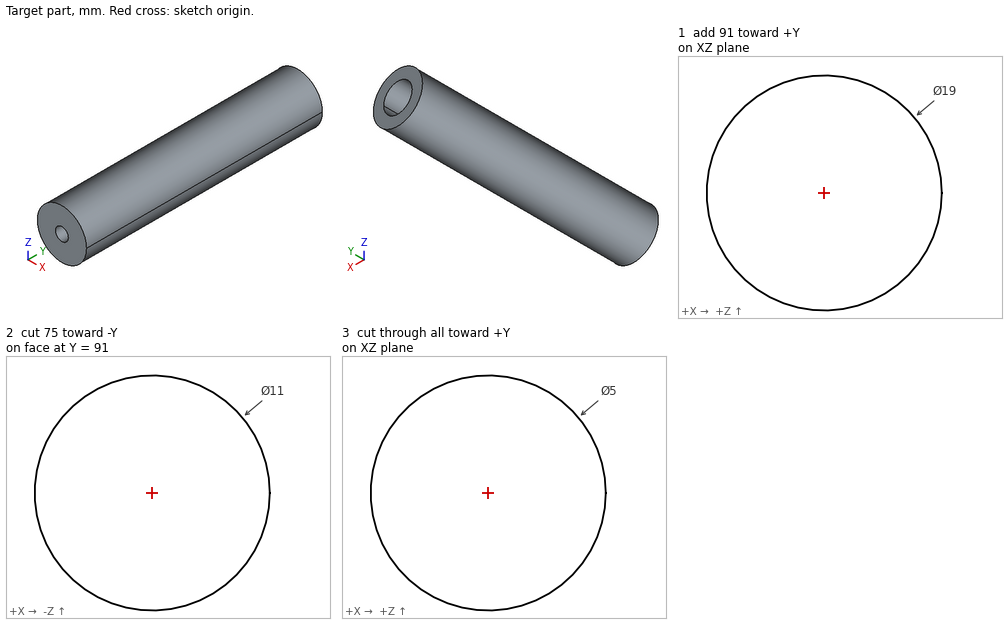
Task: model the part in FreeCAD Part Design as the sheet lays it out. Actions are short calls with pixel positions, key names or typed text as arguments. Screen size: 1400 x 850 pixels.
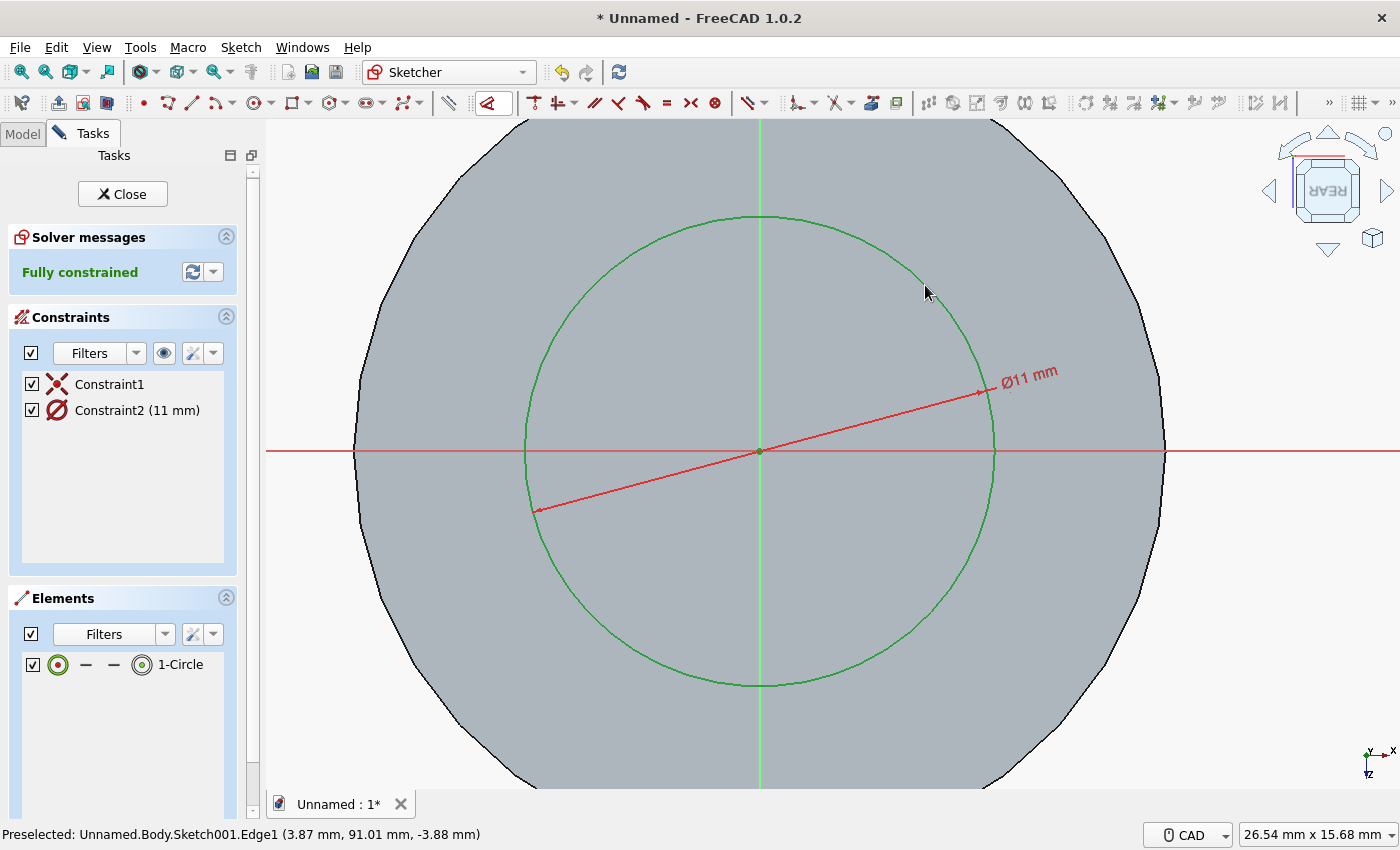
click(123, 194)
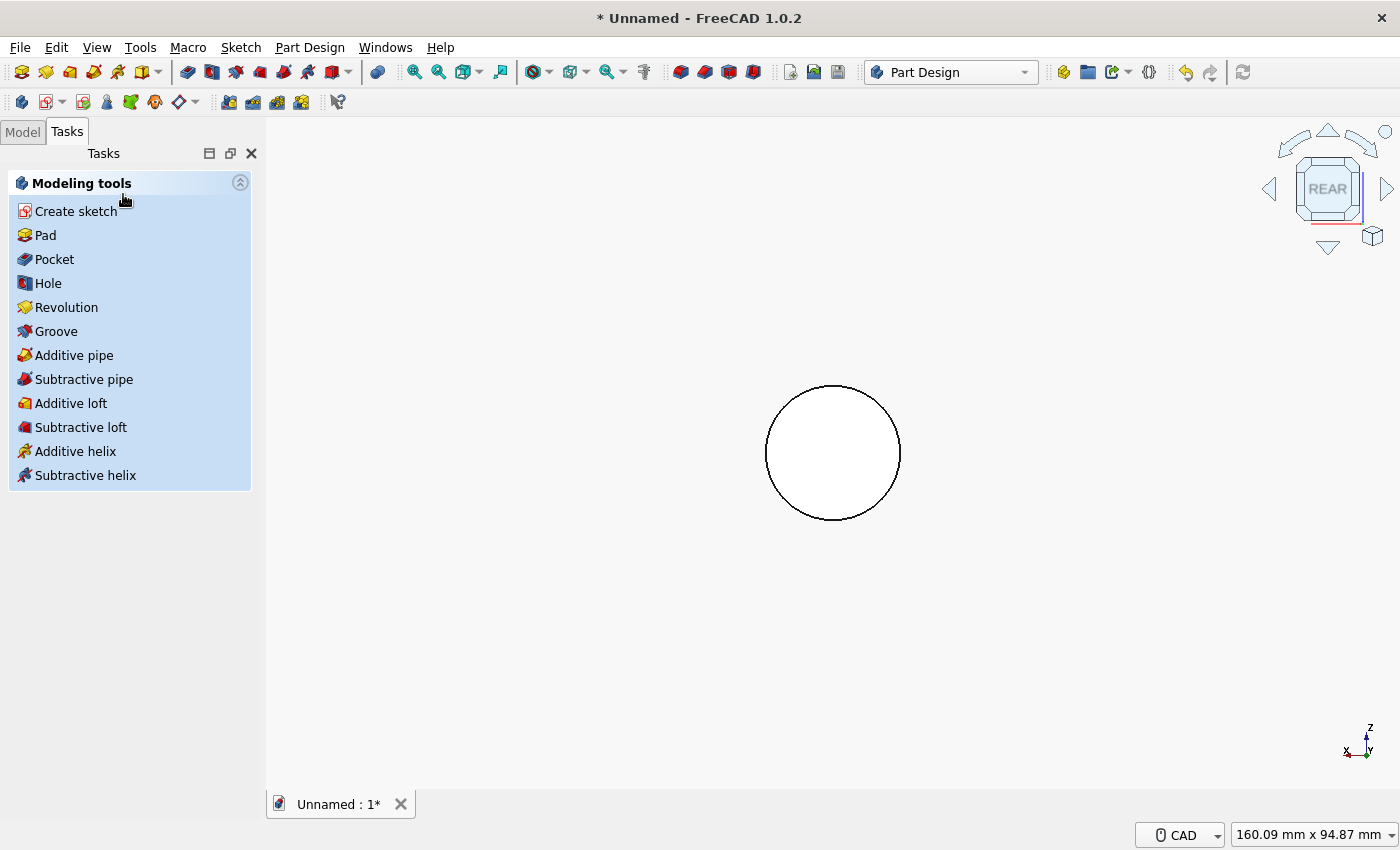
click(188, 72)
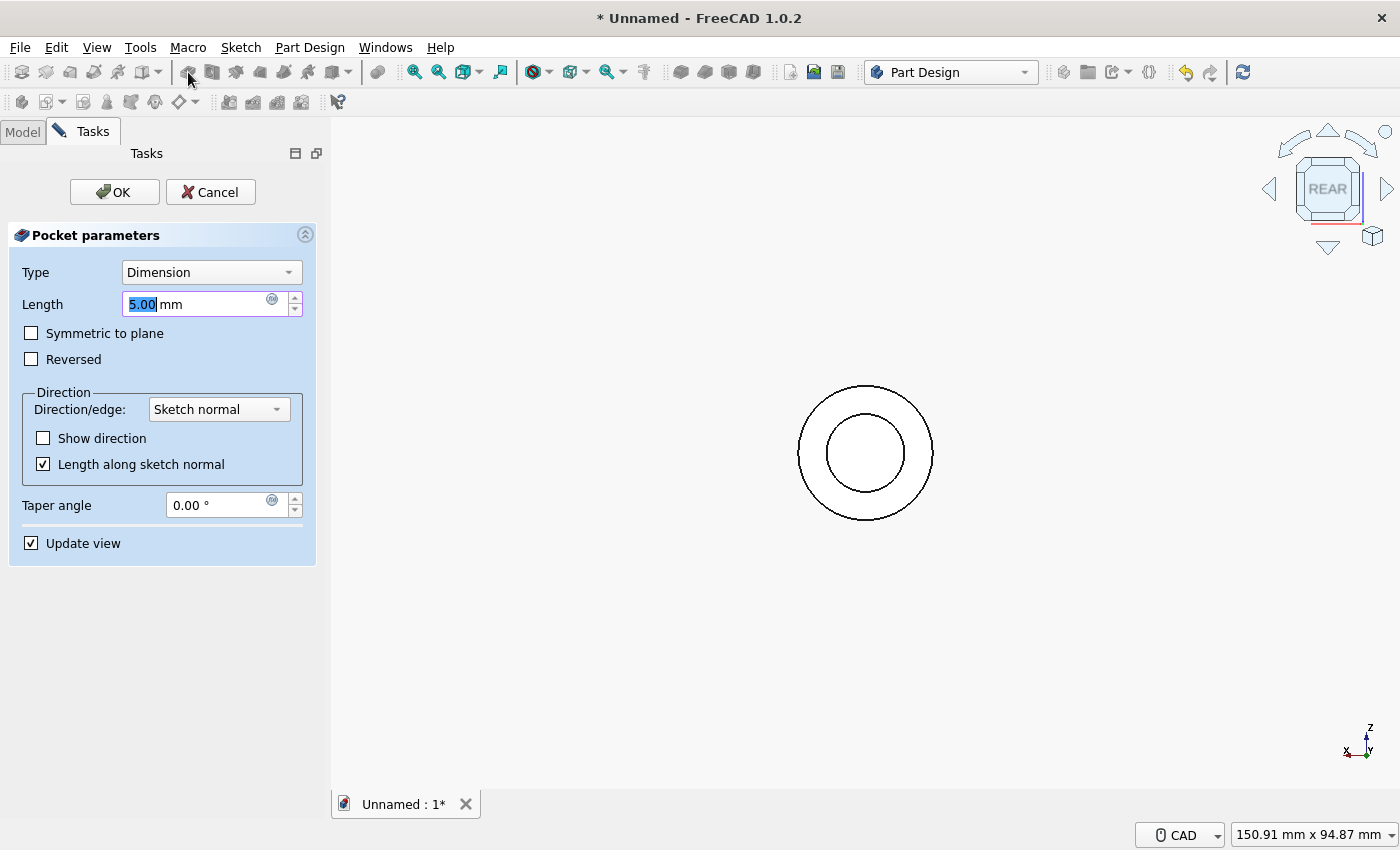
text(75)
key(Tab)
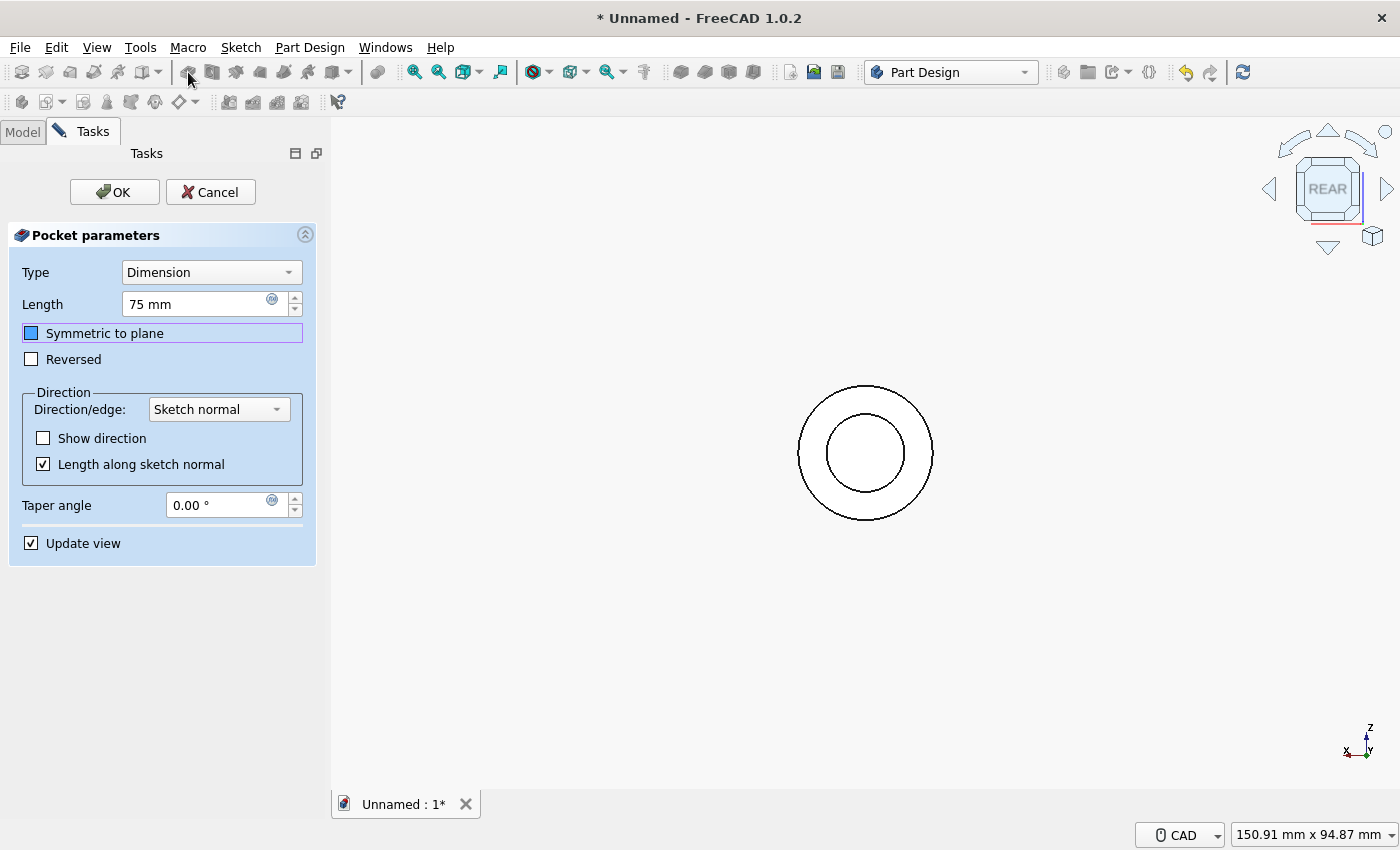
click(115, 192)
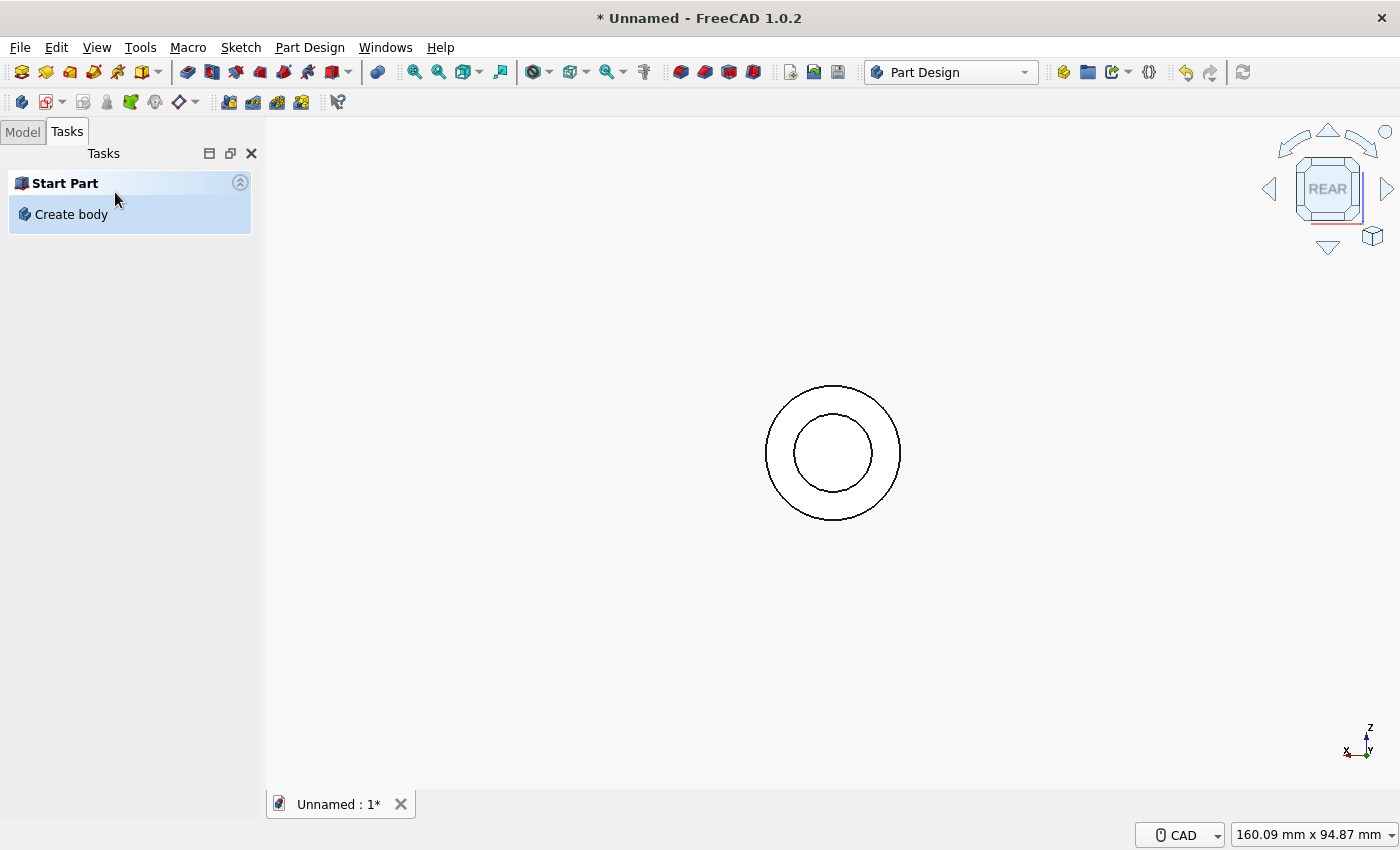
click(416, 72)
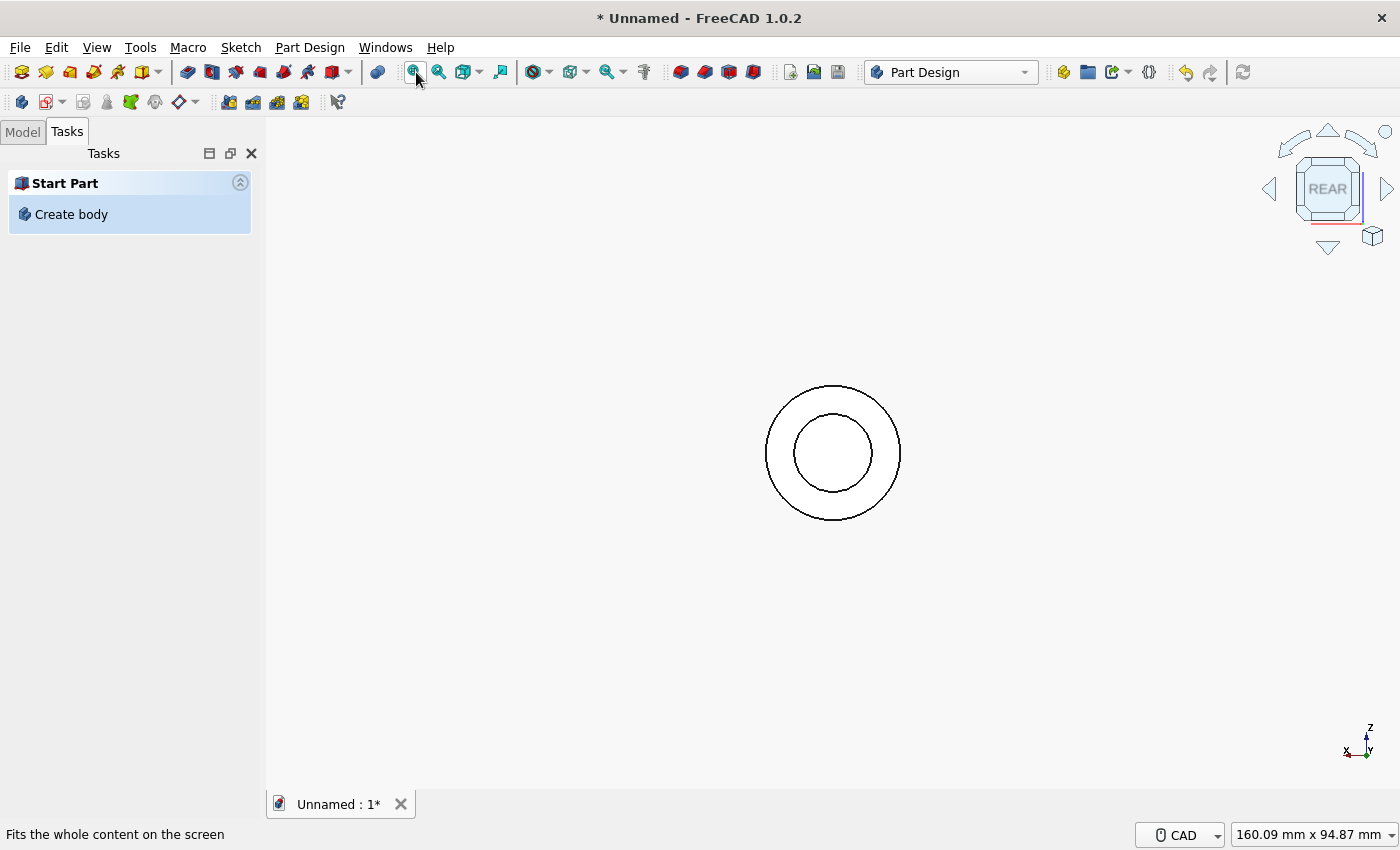
click(46, 102)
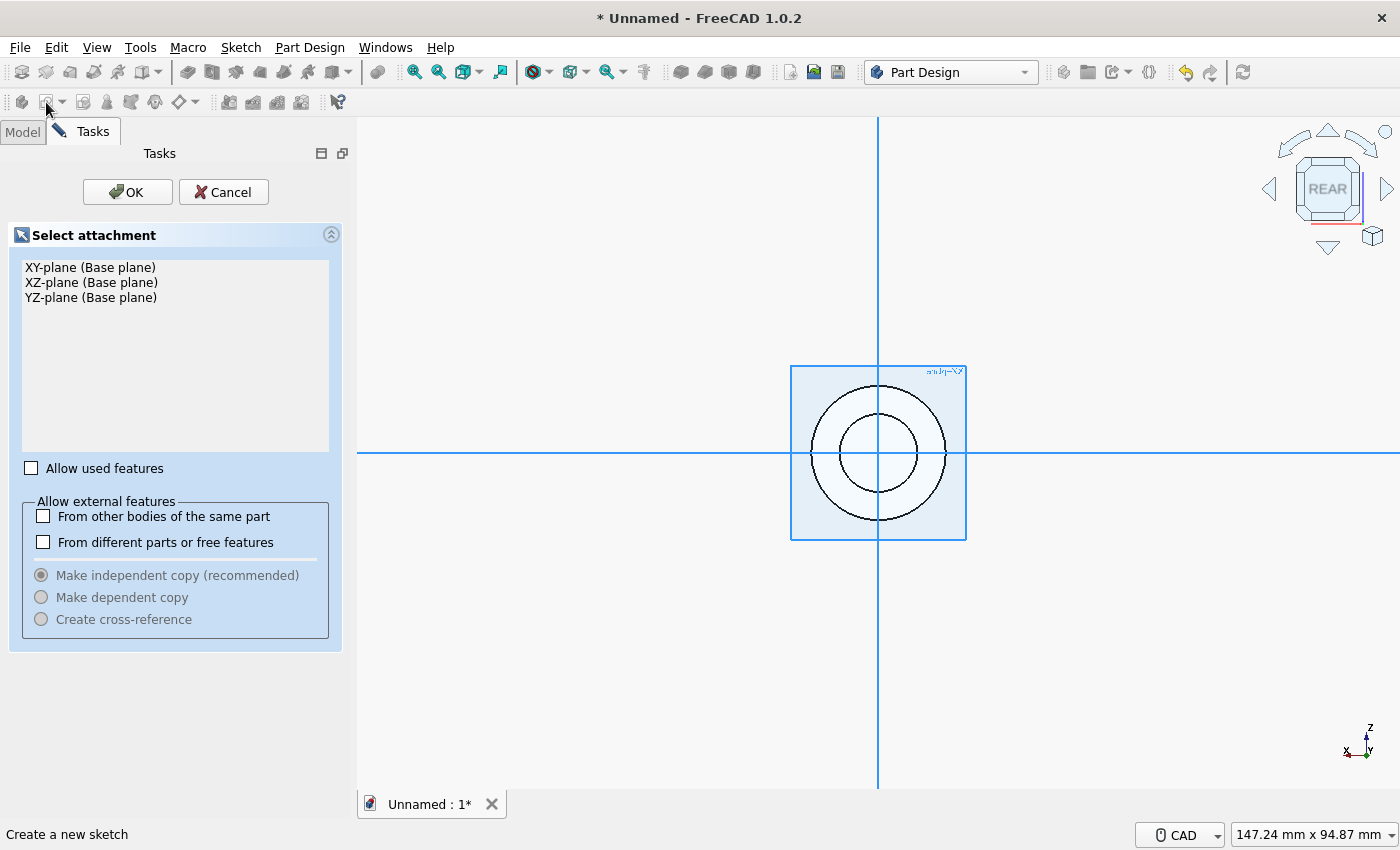
click(82, 282)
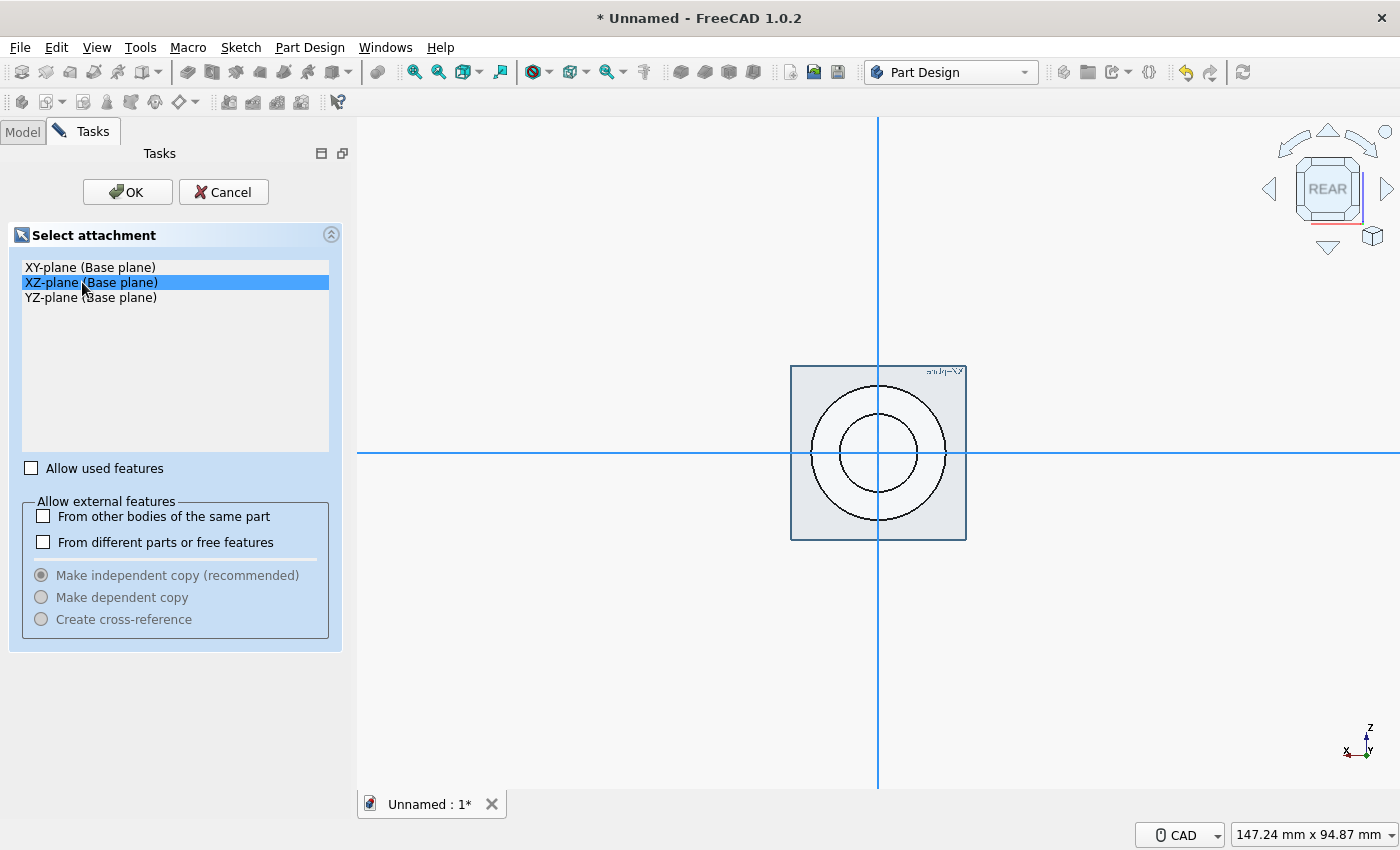
click(128, 192)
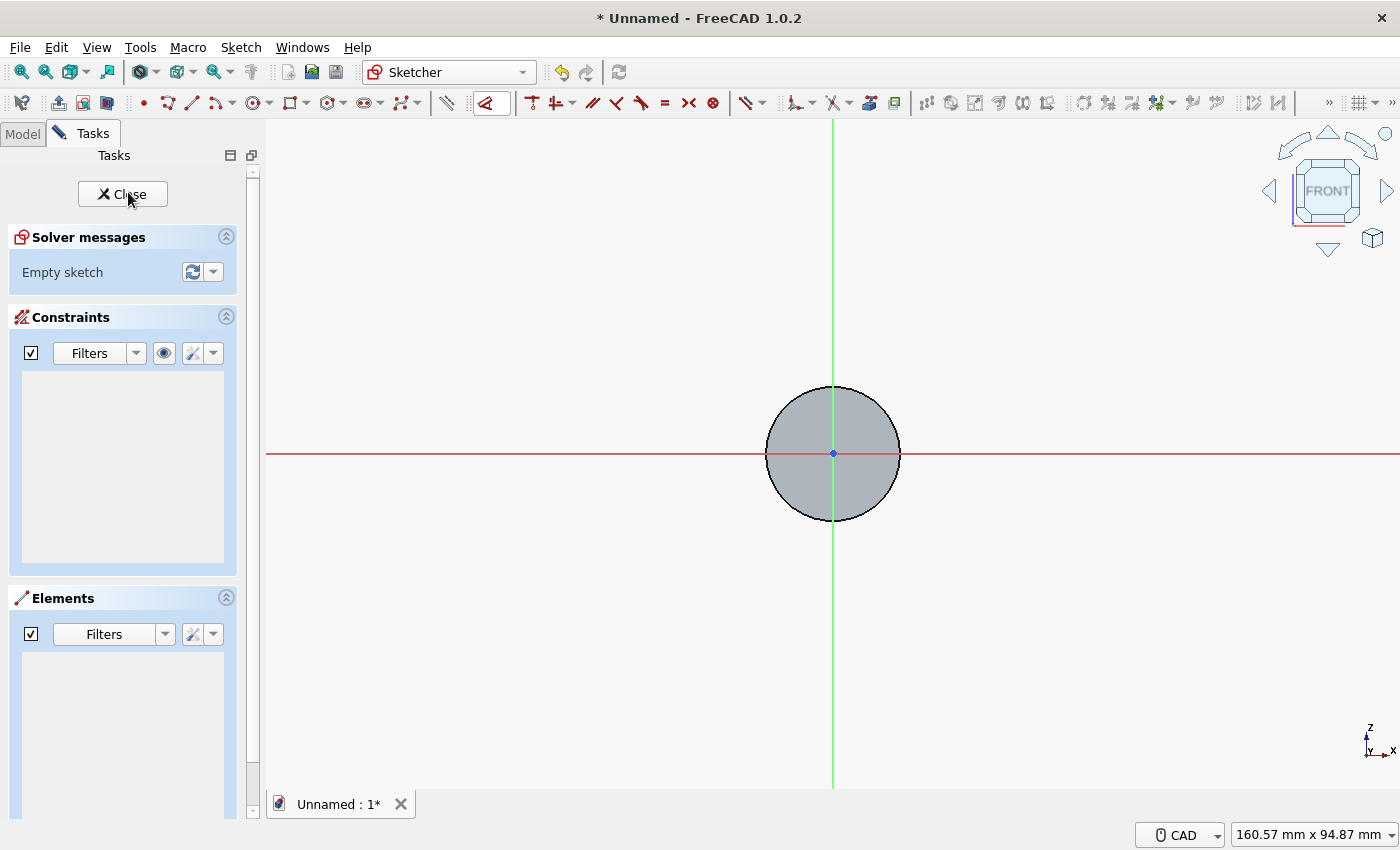
scroll(838, 454, up, 13)